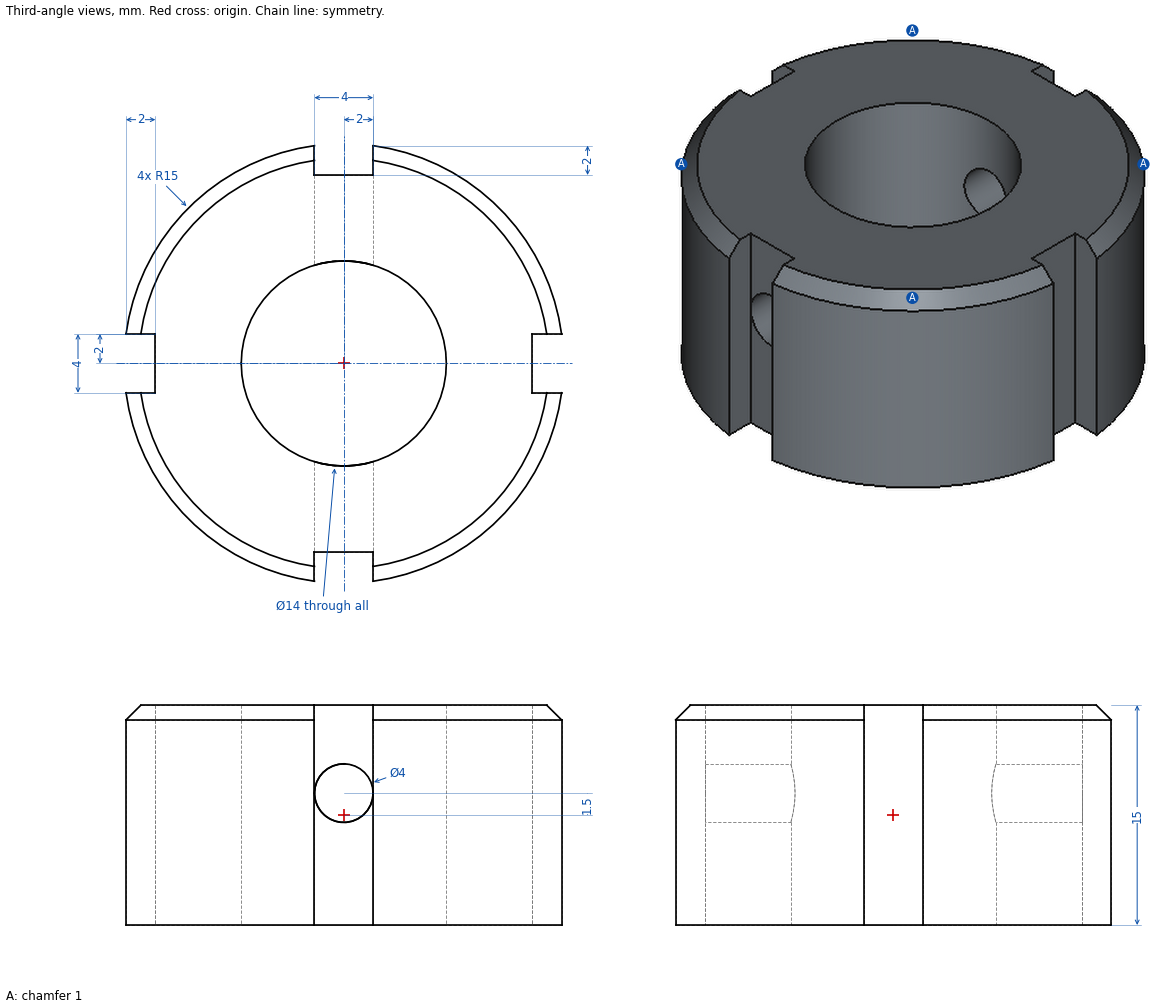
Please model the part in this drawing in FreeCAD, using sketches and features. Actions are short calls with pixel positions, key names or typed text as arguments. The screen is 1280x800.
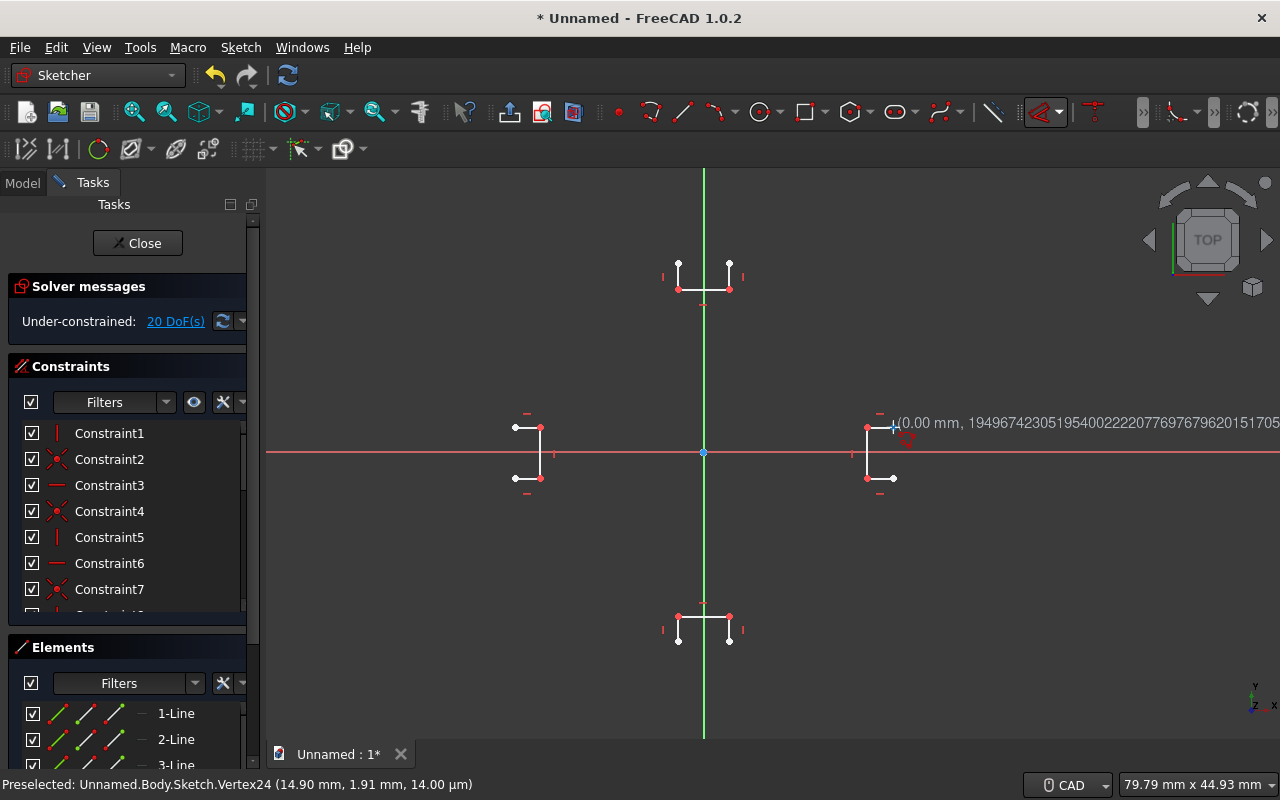
click(716, 112)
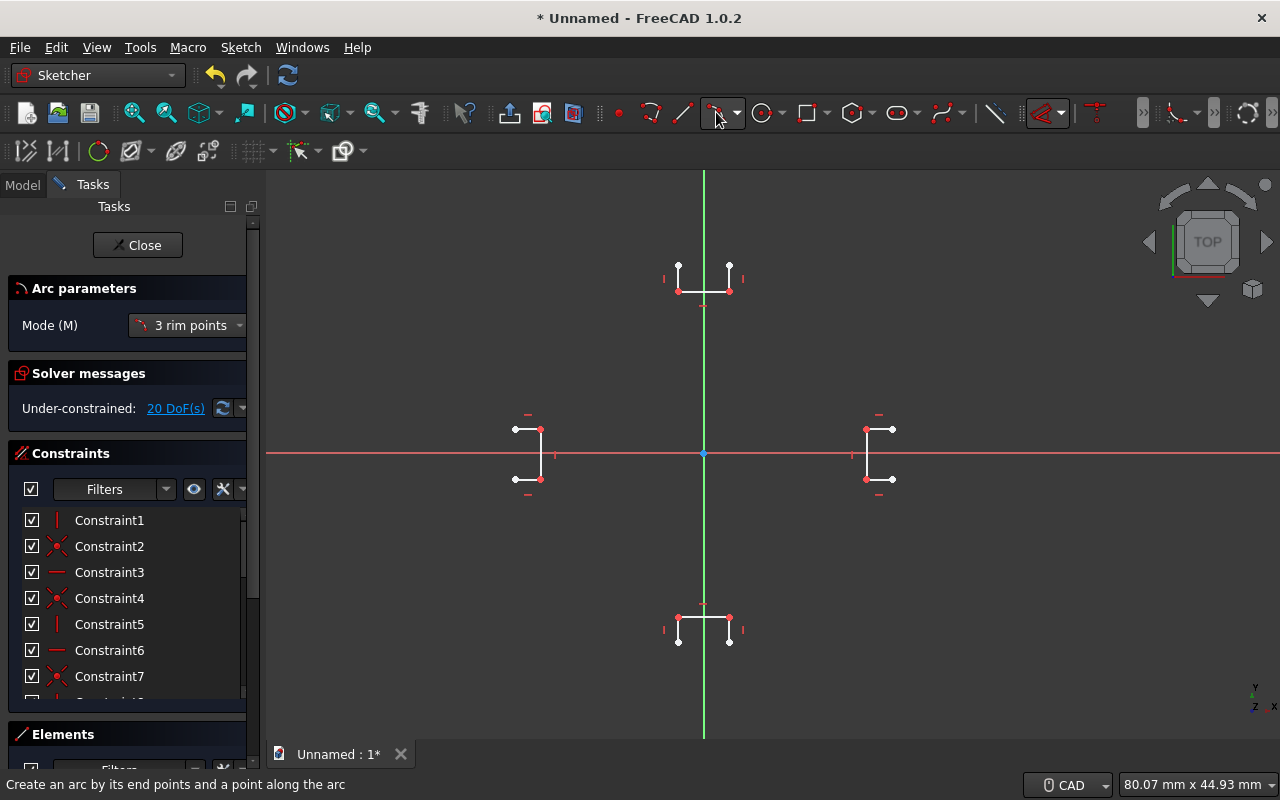
scroll(679, 265, up, 2)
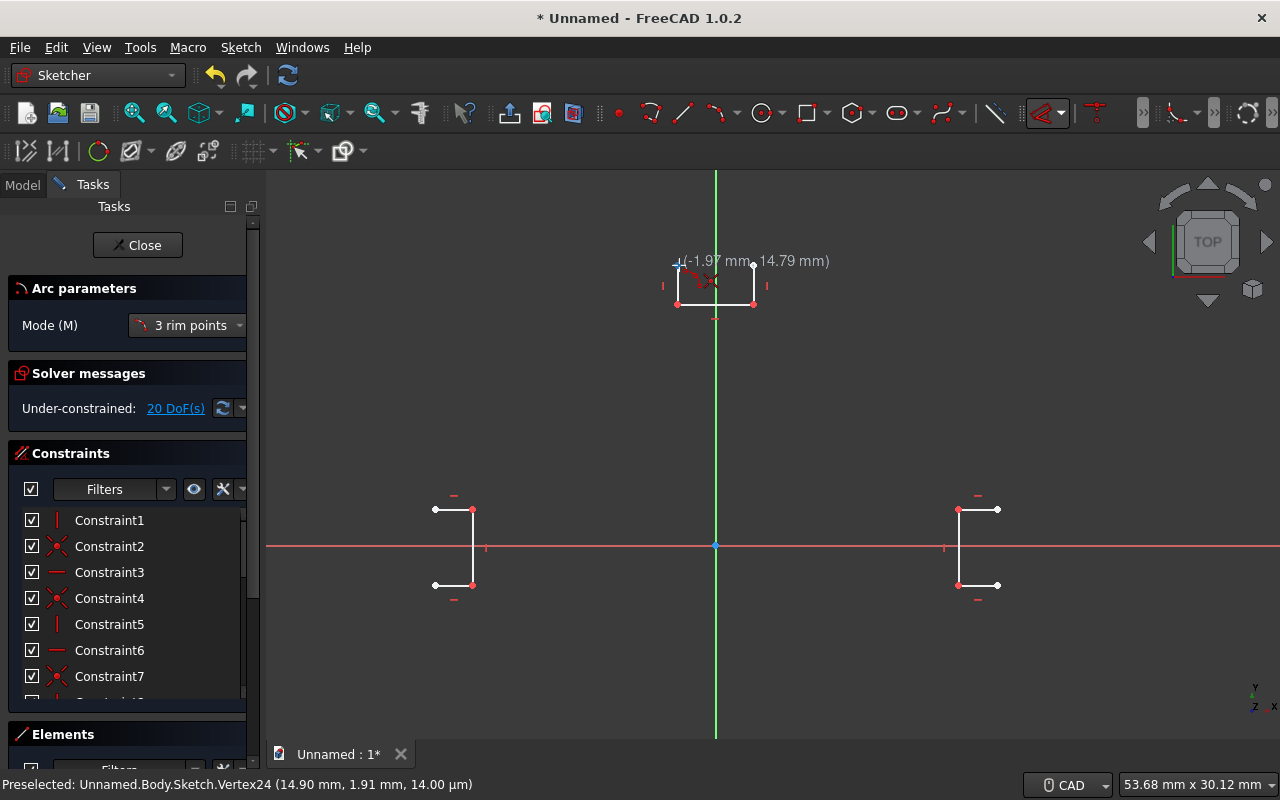
click(678, 266)
click(435, 510)
click(516, 345)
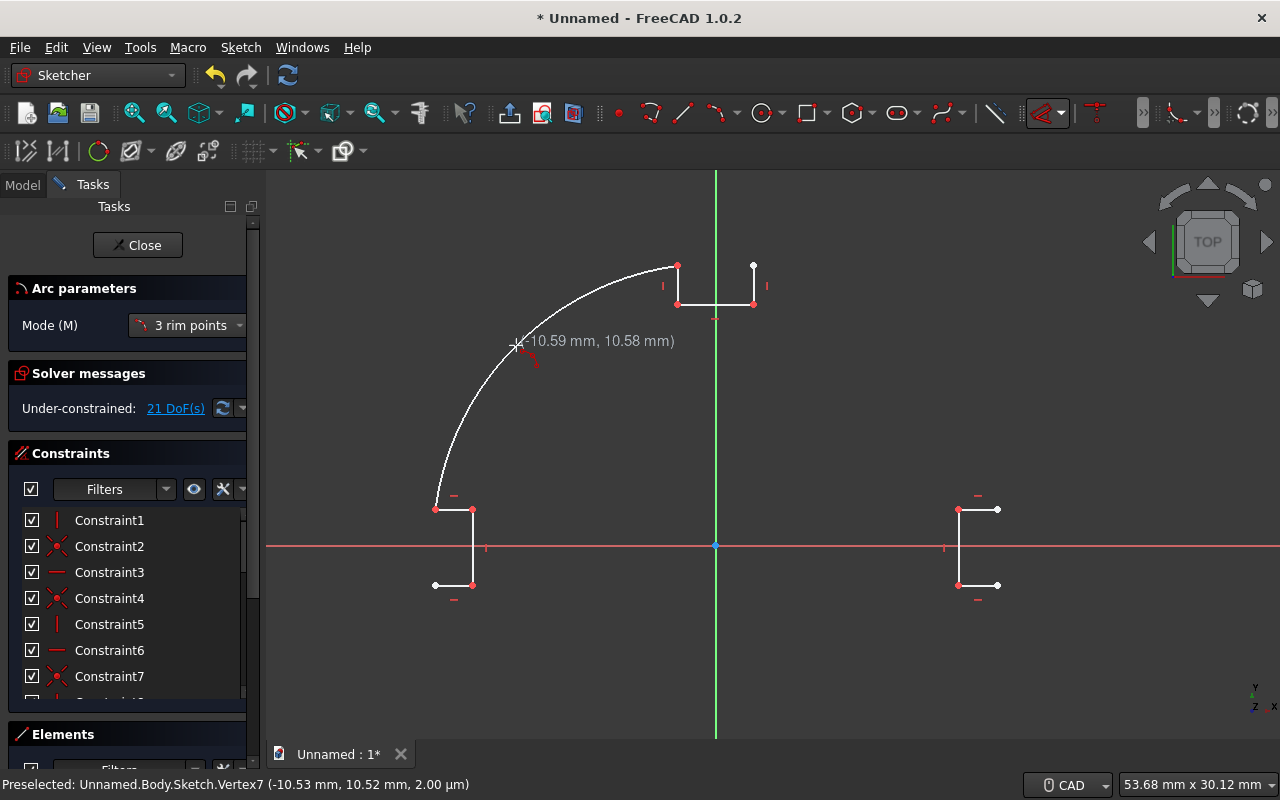
click(435, 586)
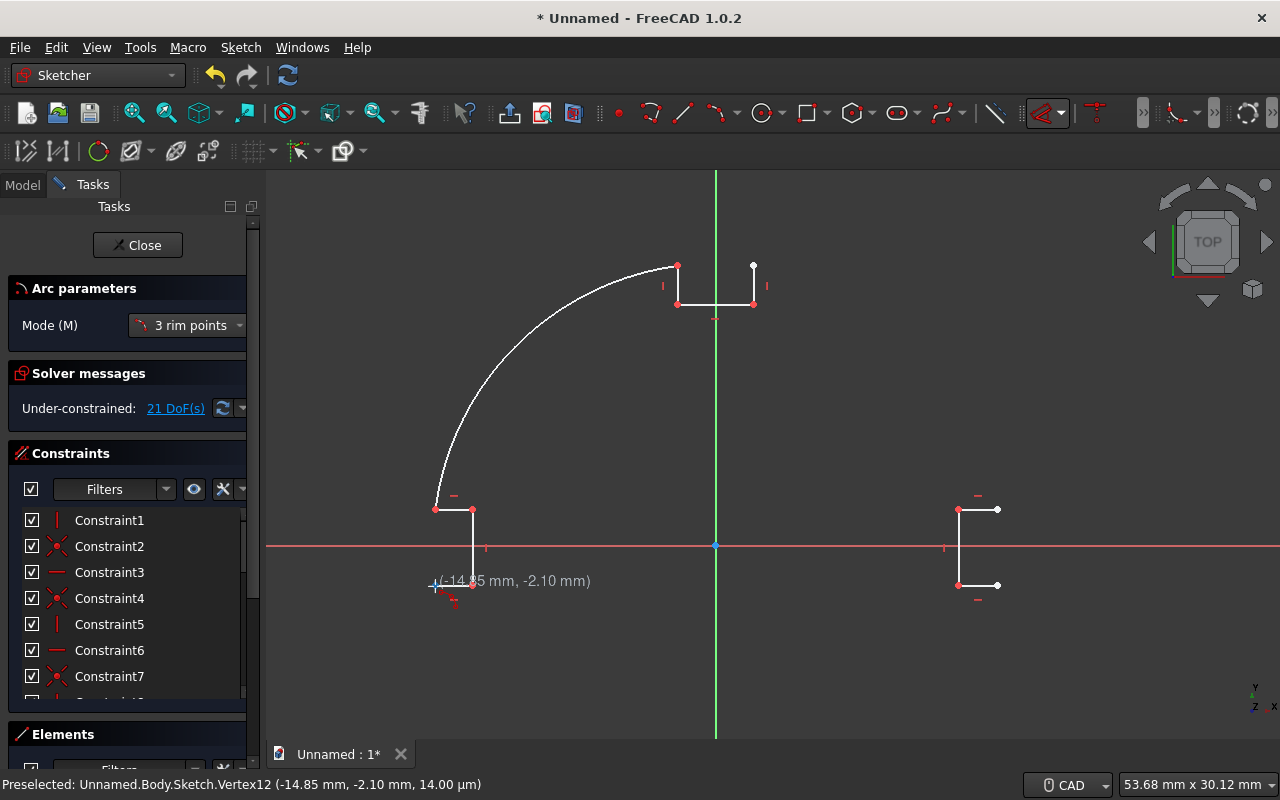
scroll(681, 269, down, 2)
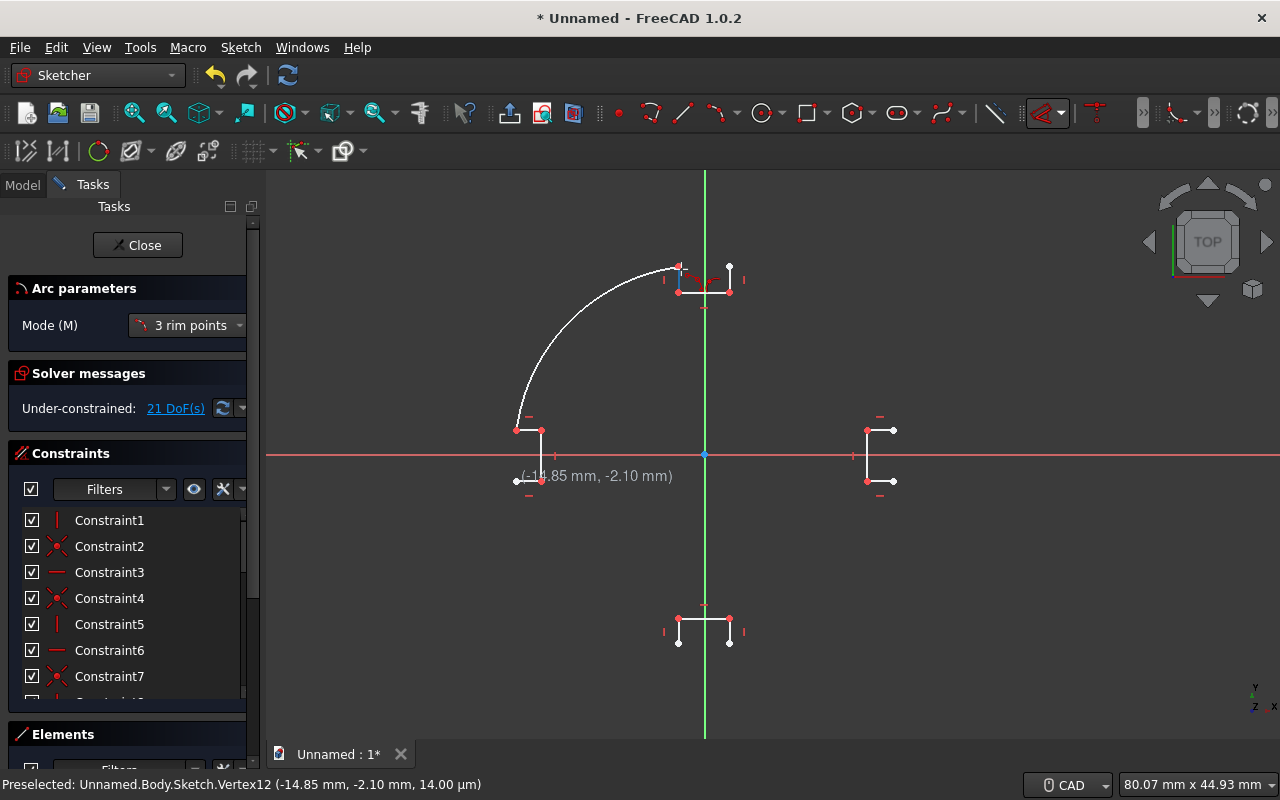
scroll(679, 643, up, 2)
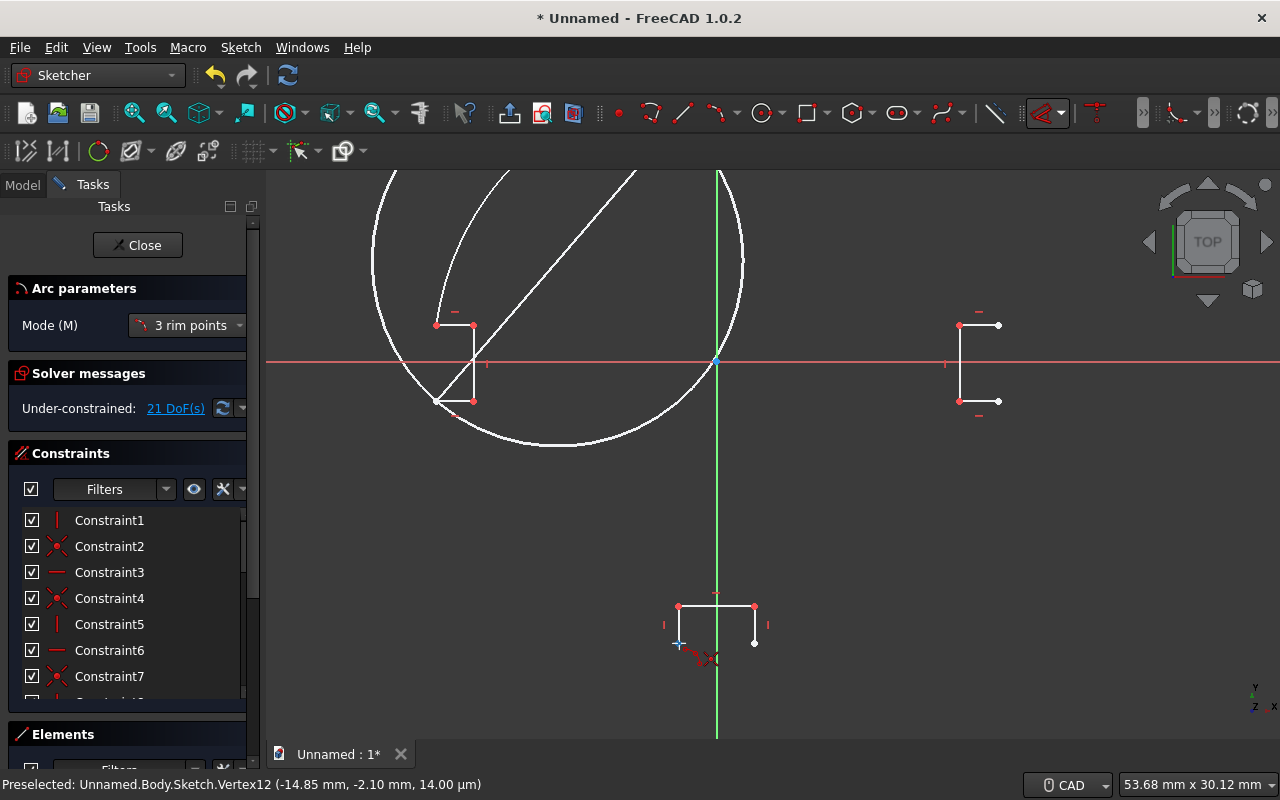
click(679, 644)
click(517, 562)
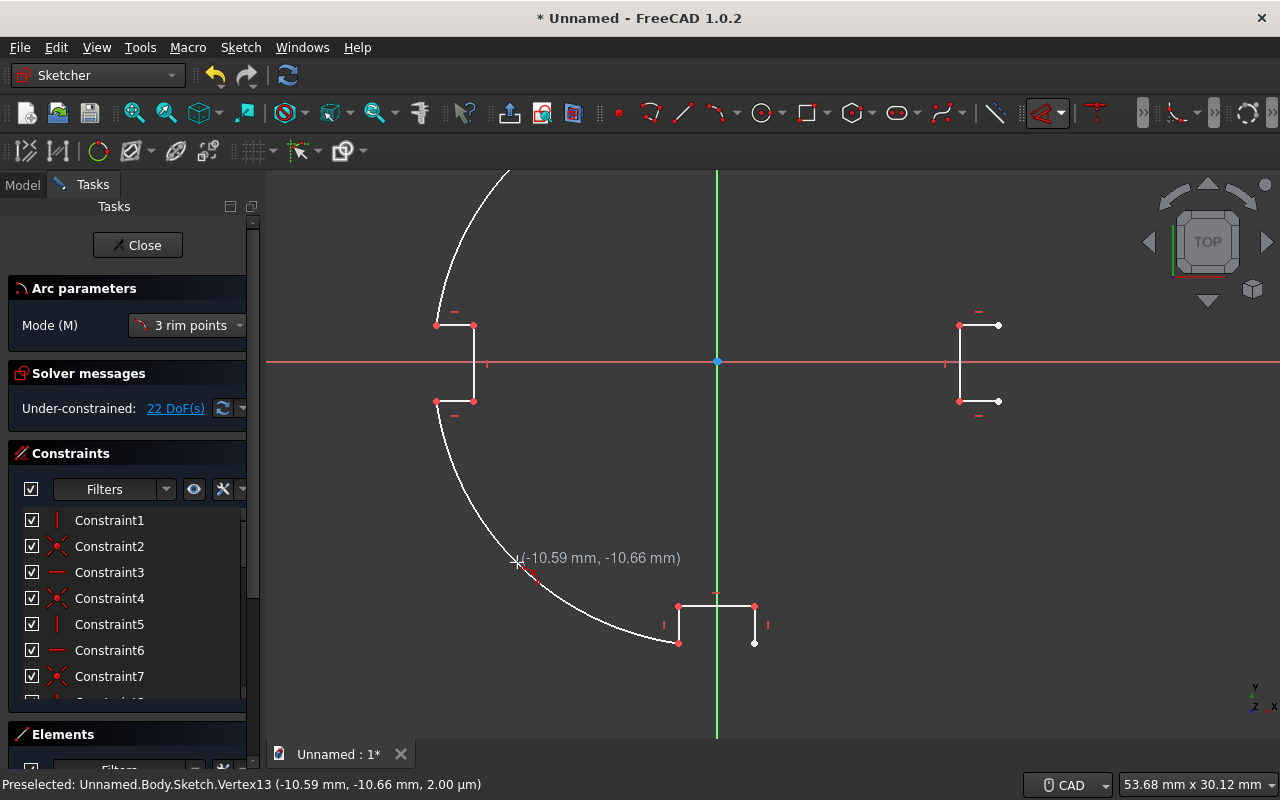
click(755, 644)
click(998, 401)
click(917, 562)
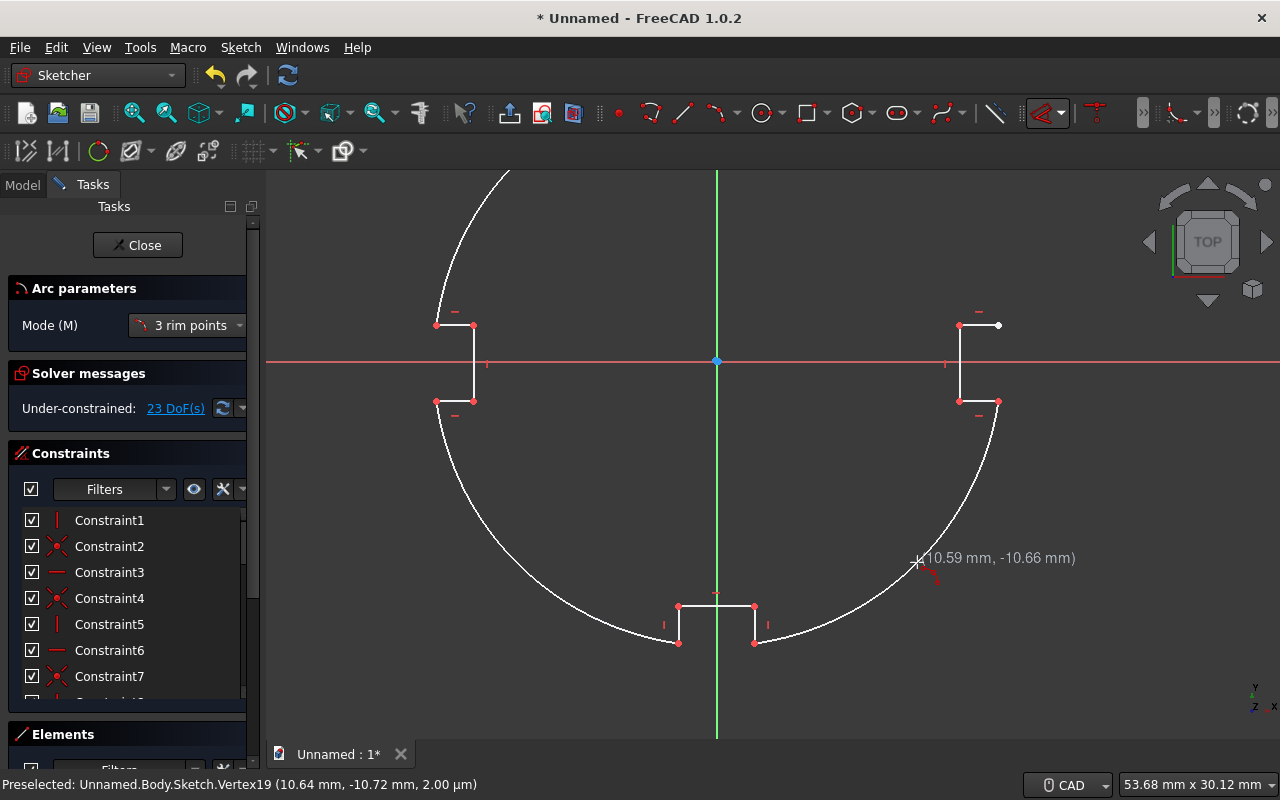
click(998, 325)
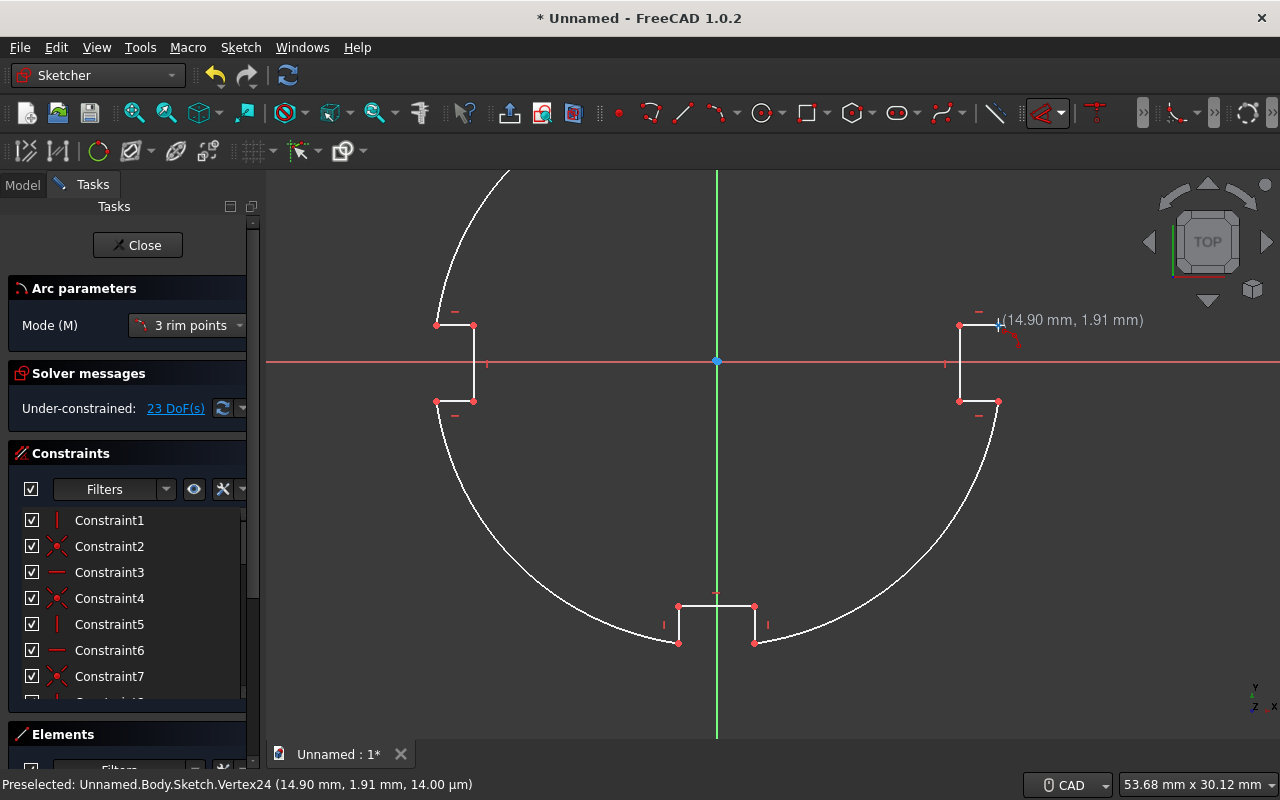
scroll(679, 644, down, 2)